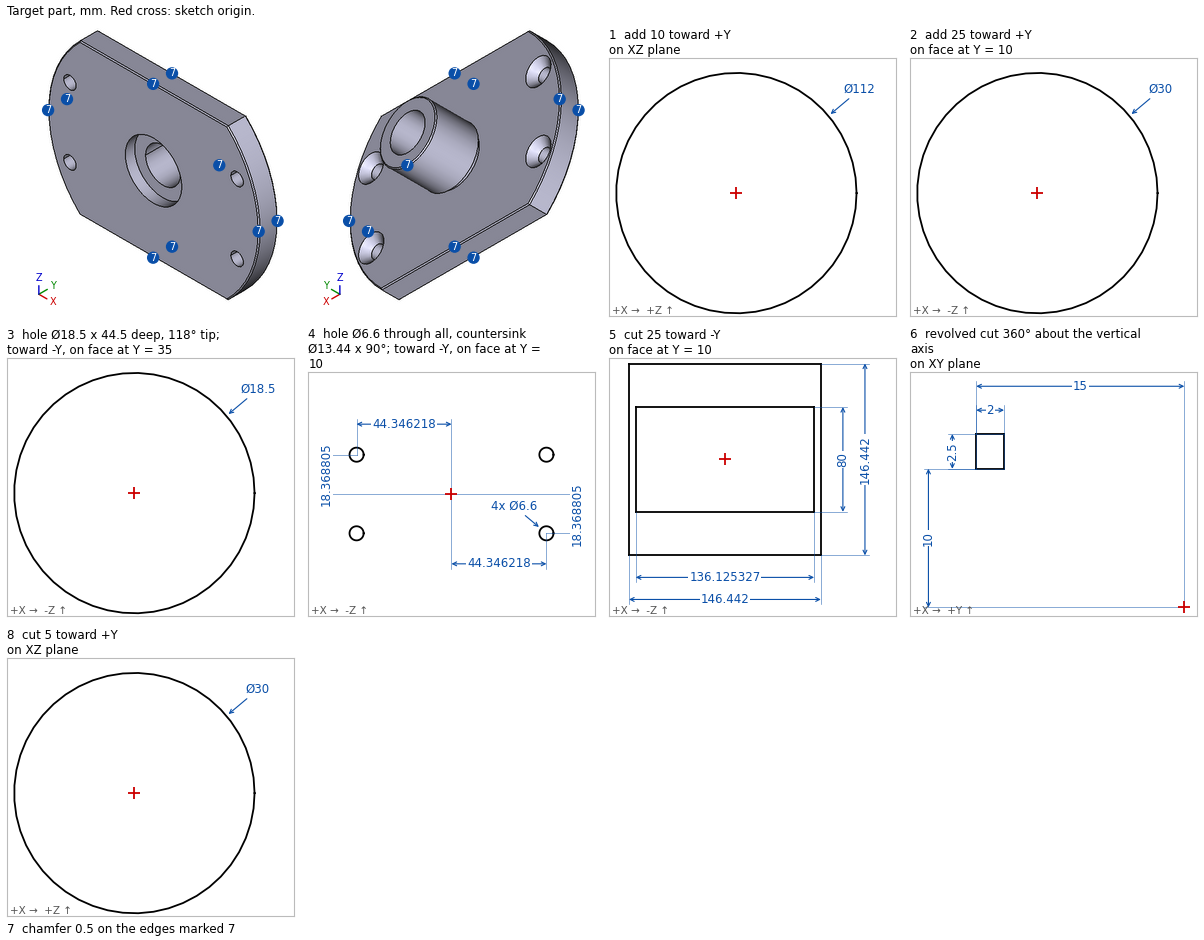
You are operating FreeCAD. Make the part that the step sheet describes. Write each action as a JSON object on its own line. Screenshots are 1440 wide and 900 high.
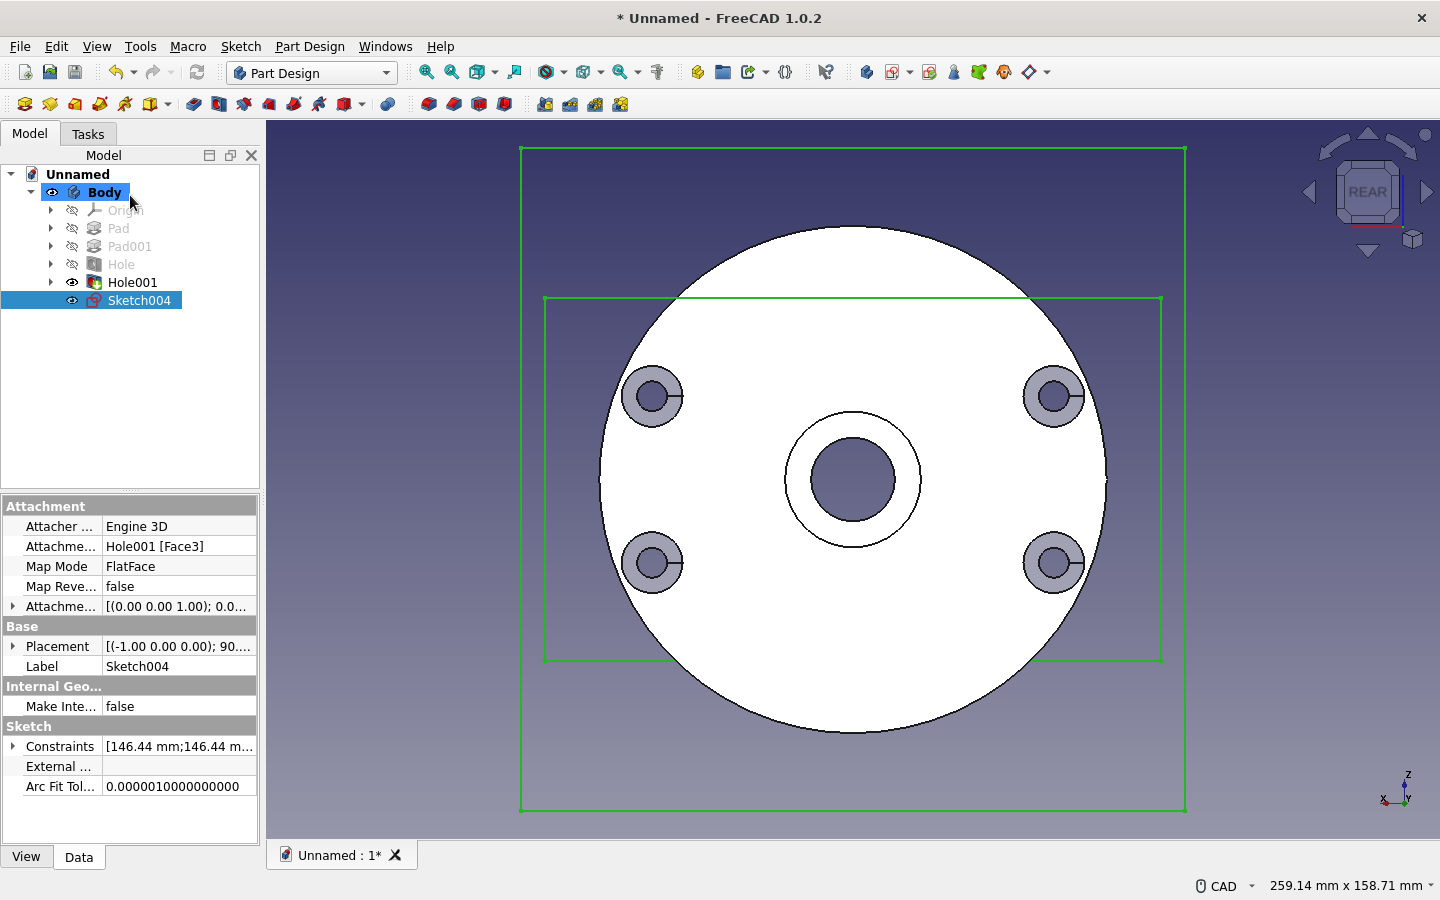
{"action": "left_click", "coordinate": [194, 104]}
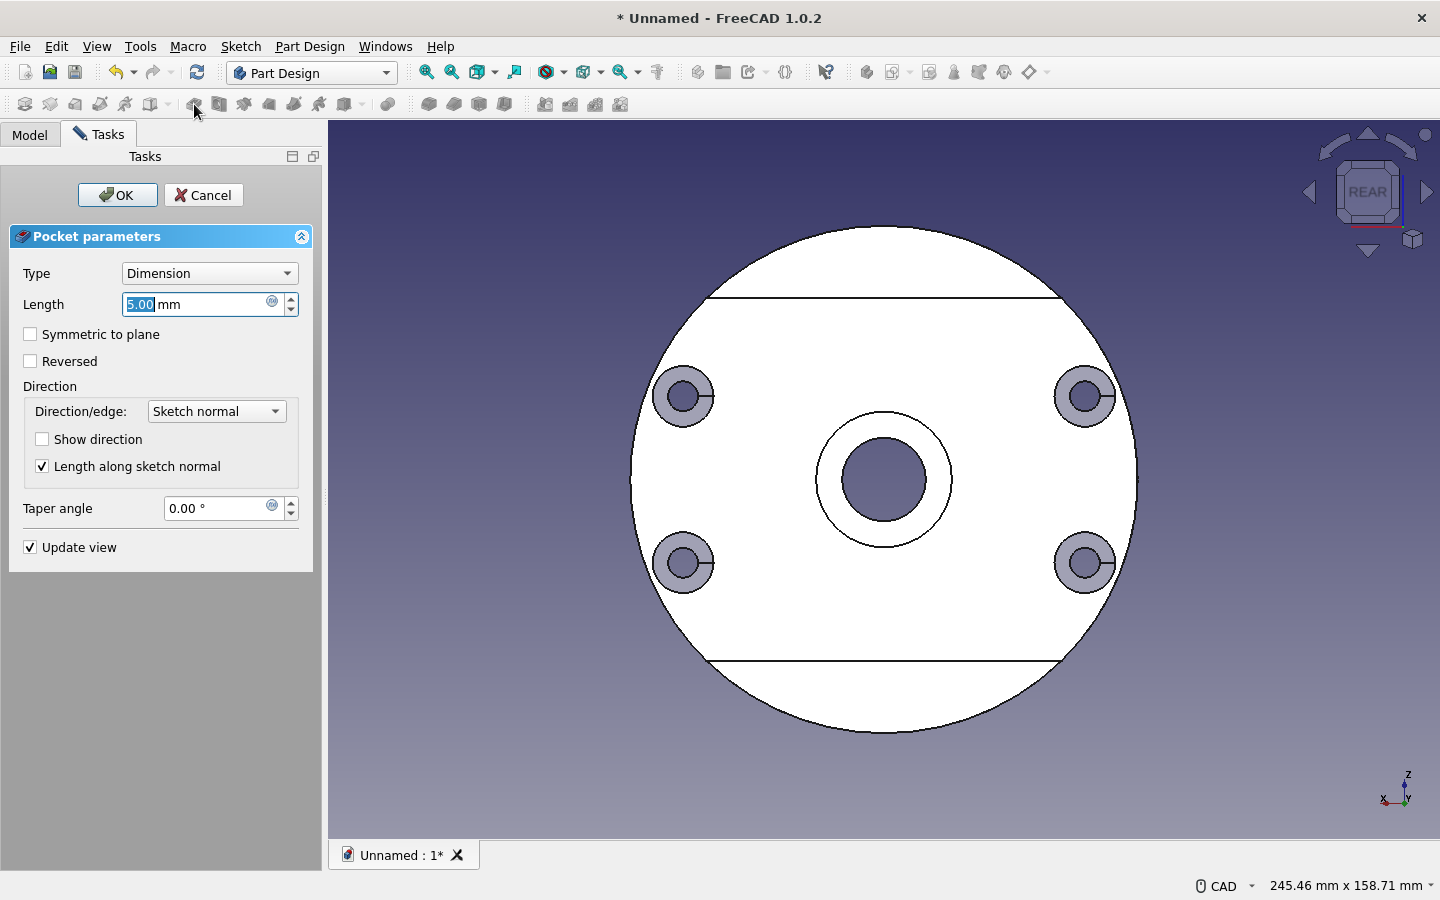
{"action": "type", "text": "25"}
{"action": "key", "text": "Tab"}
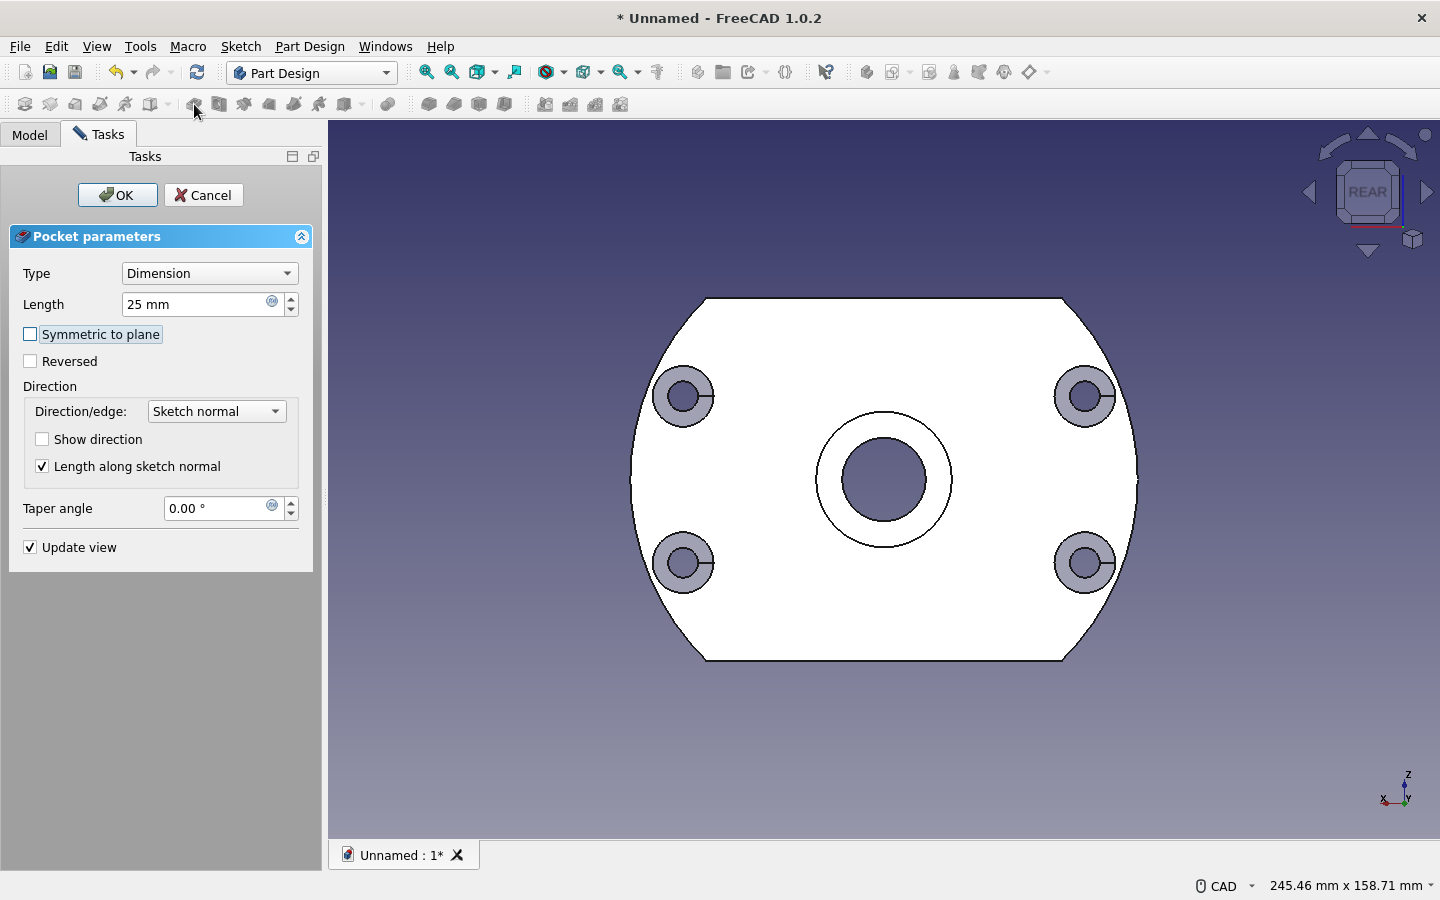
{"action": "left_click", "coordinate": [118, 195]}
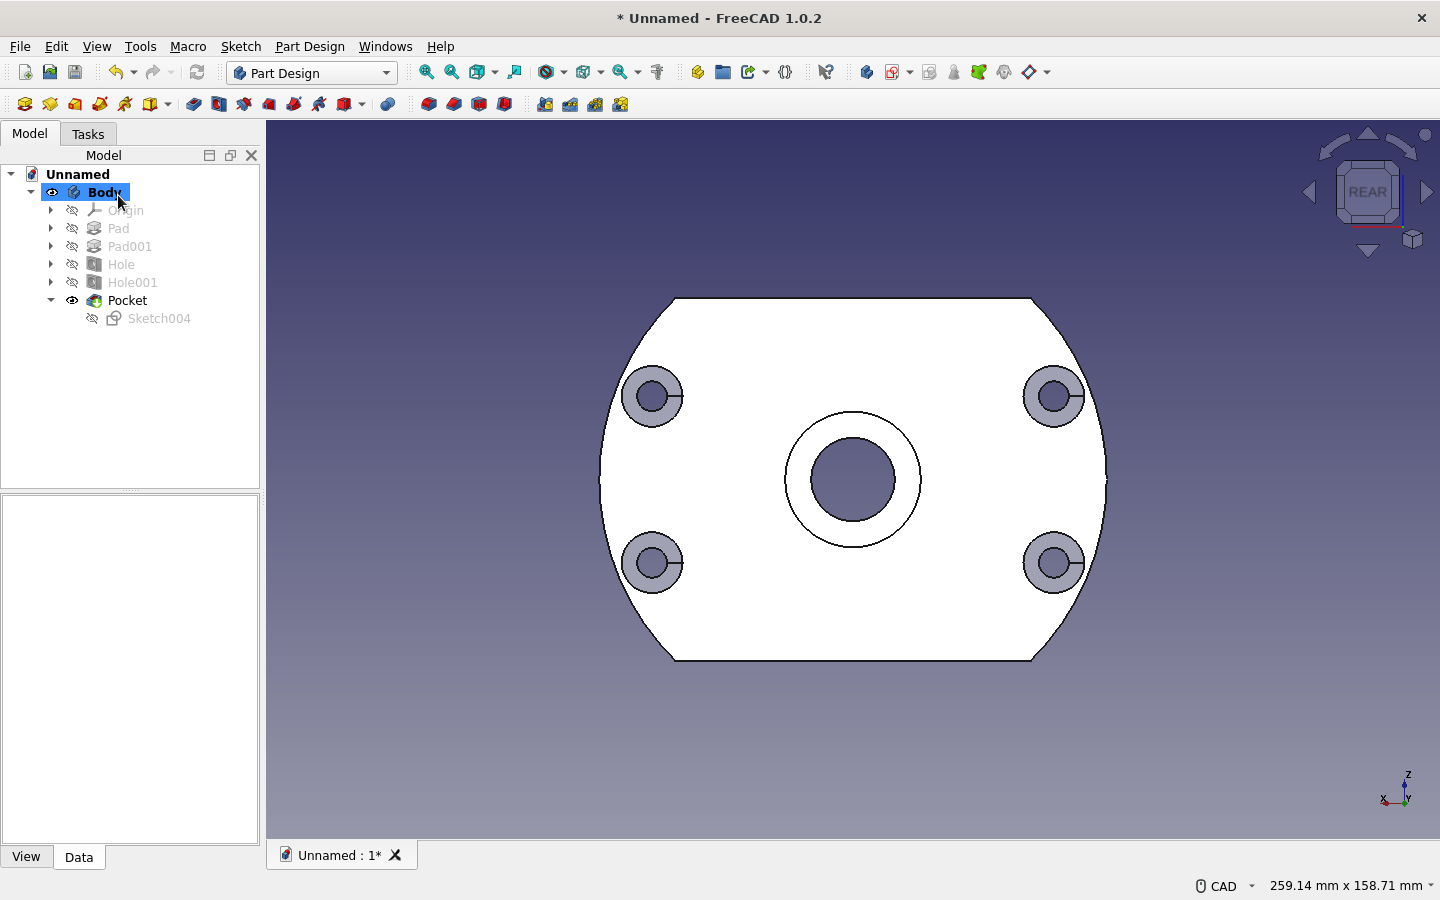
{"action": "left_click", "coordinate": [892, 72]}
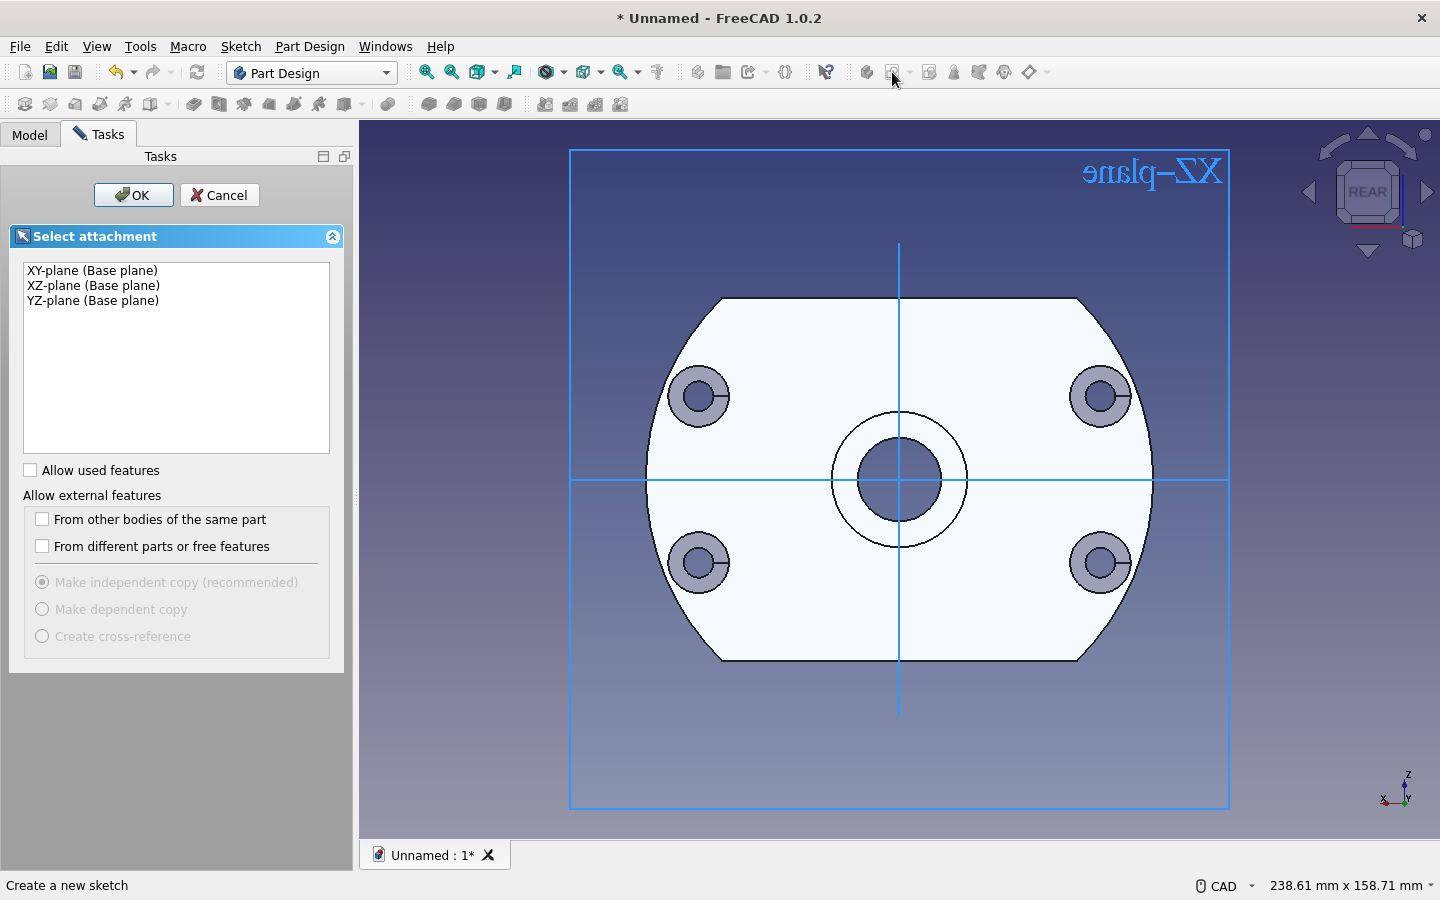
{"action": "left_click", "coordinate": [84, 270]}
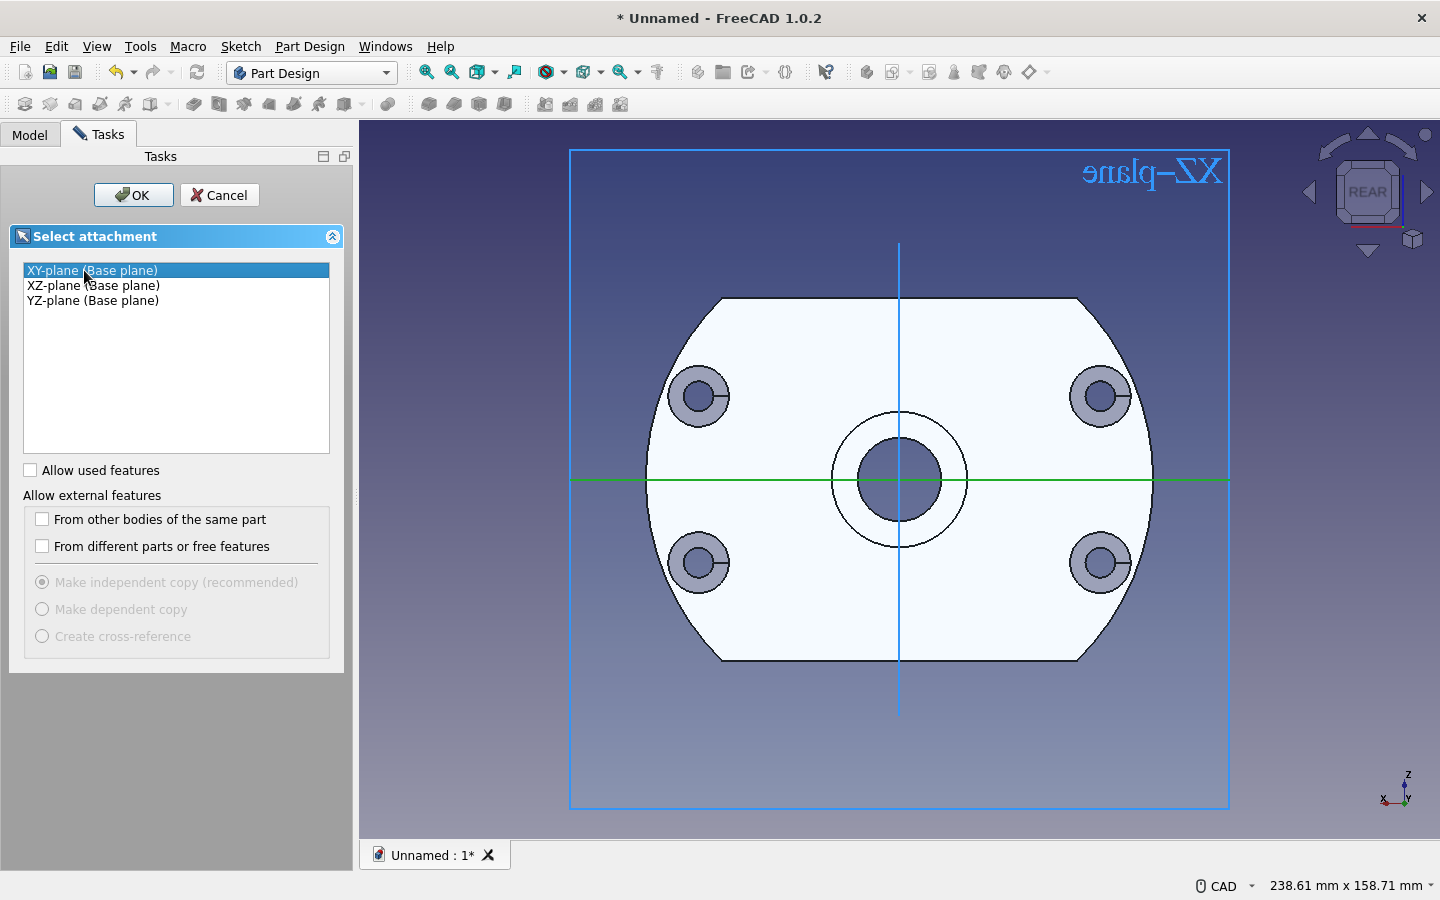
{"action": "left_click", "coordinate": [134, 195]}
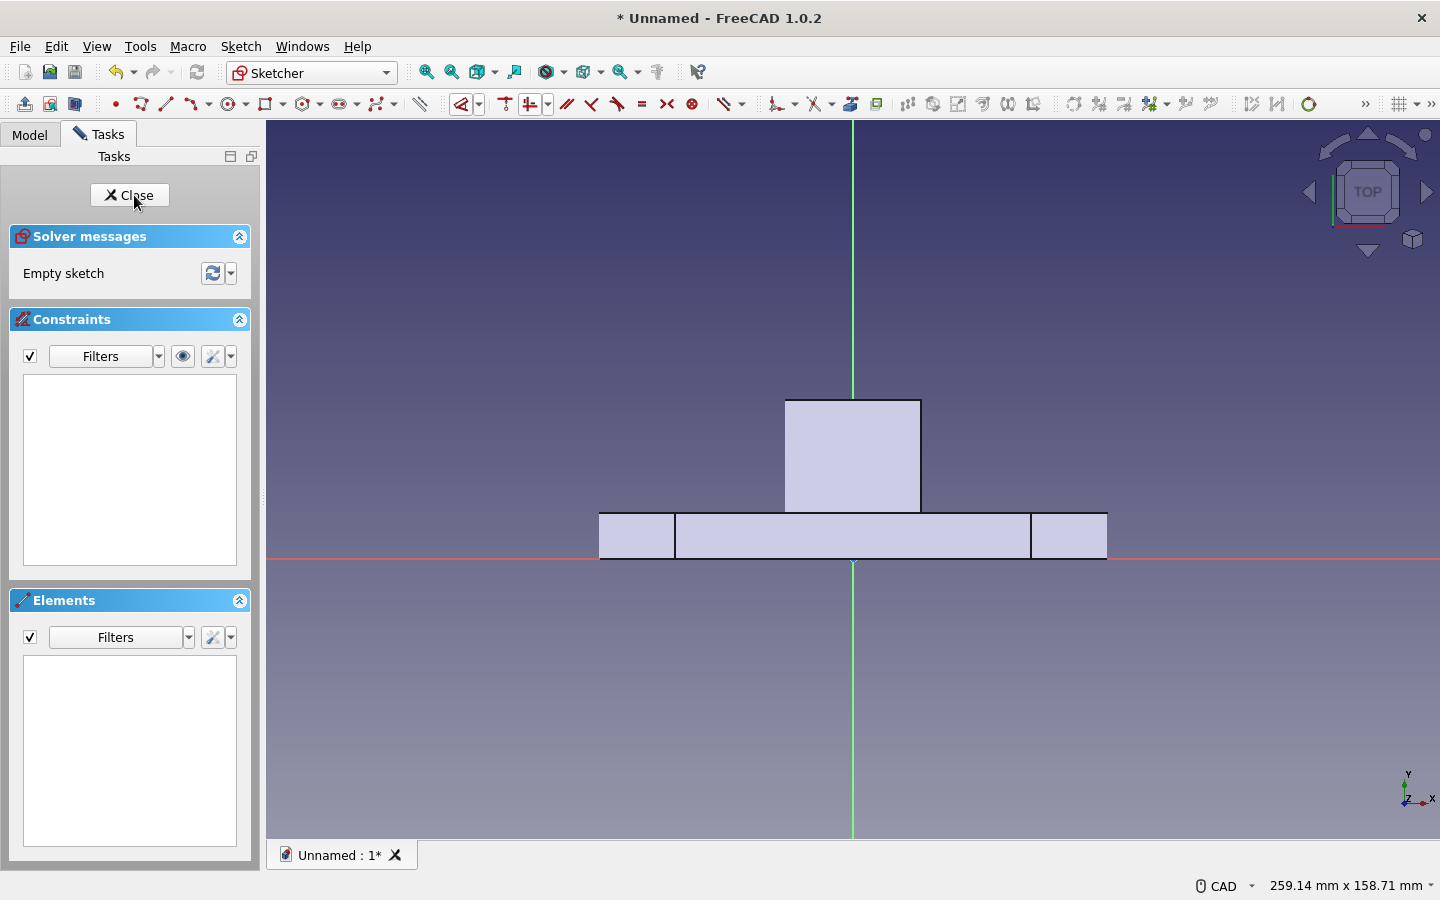
{"action": "key", "text": "q s"}